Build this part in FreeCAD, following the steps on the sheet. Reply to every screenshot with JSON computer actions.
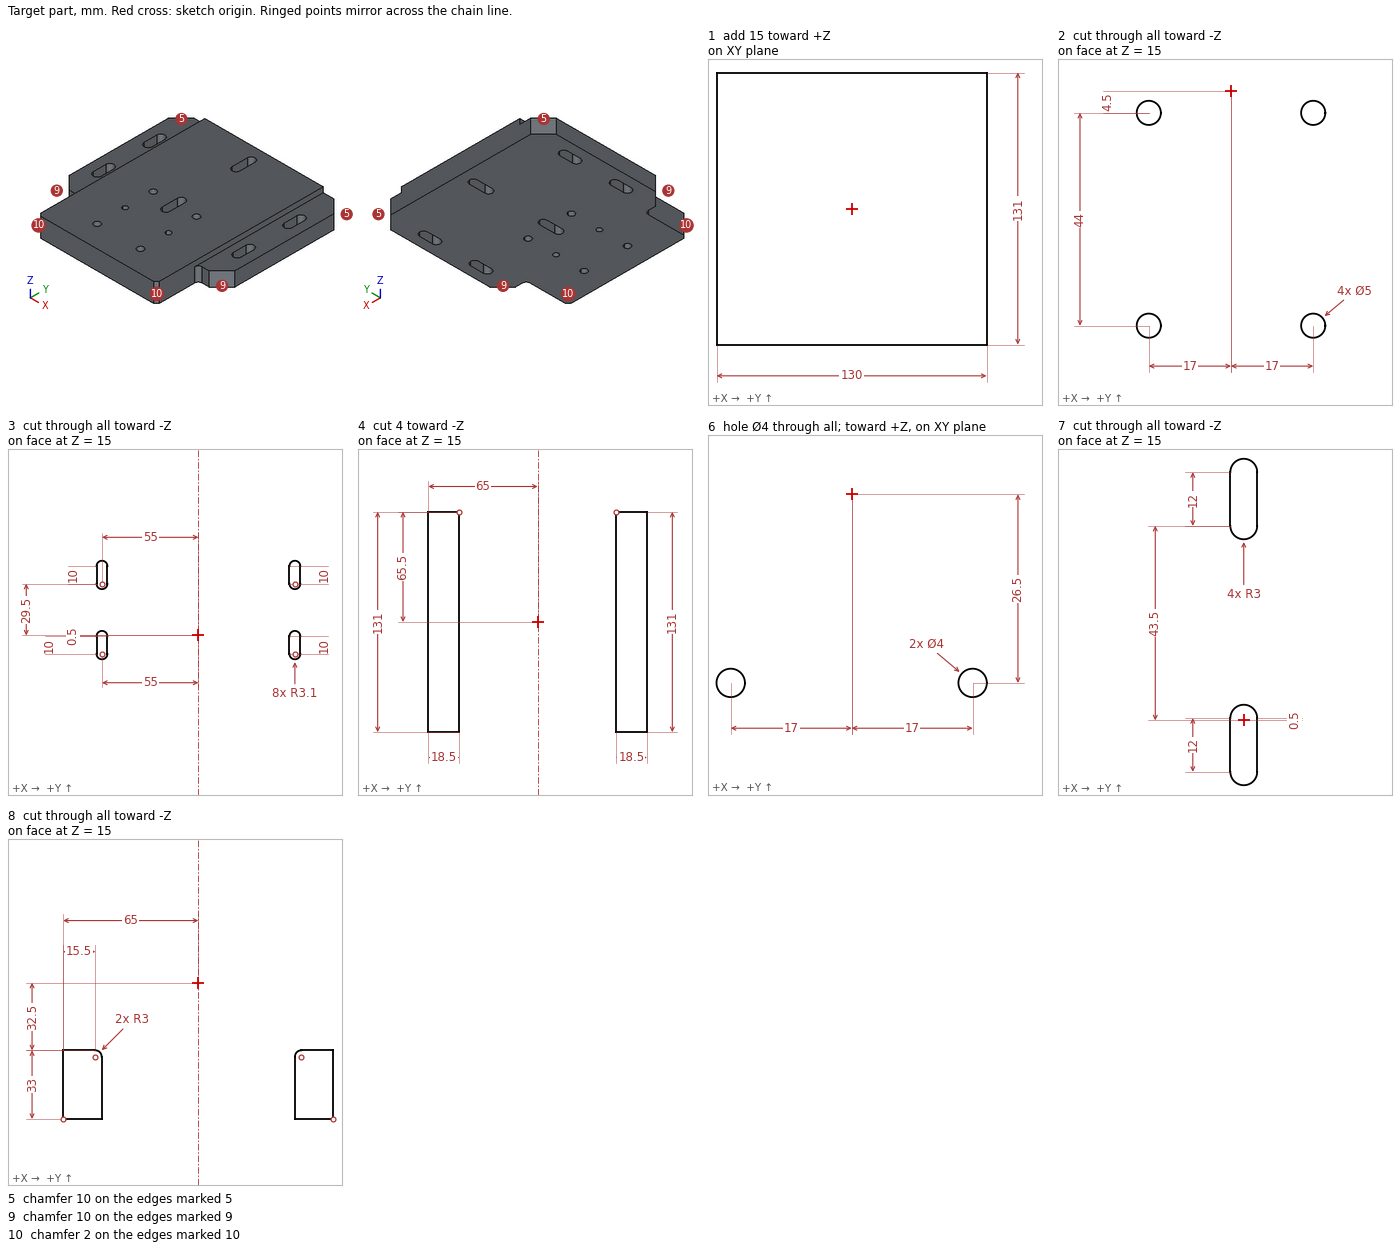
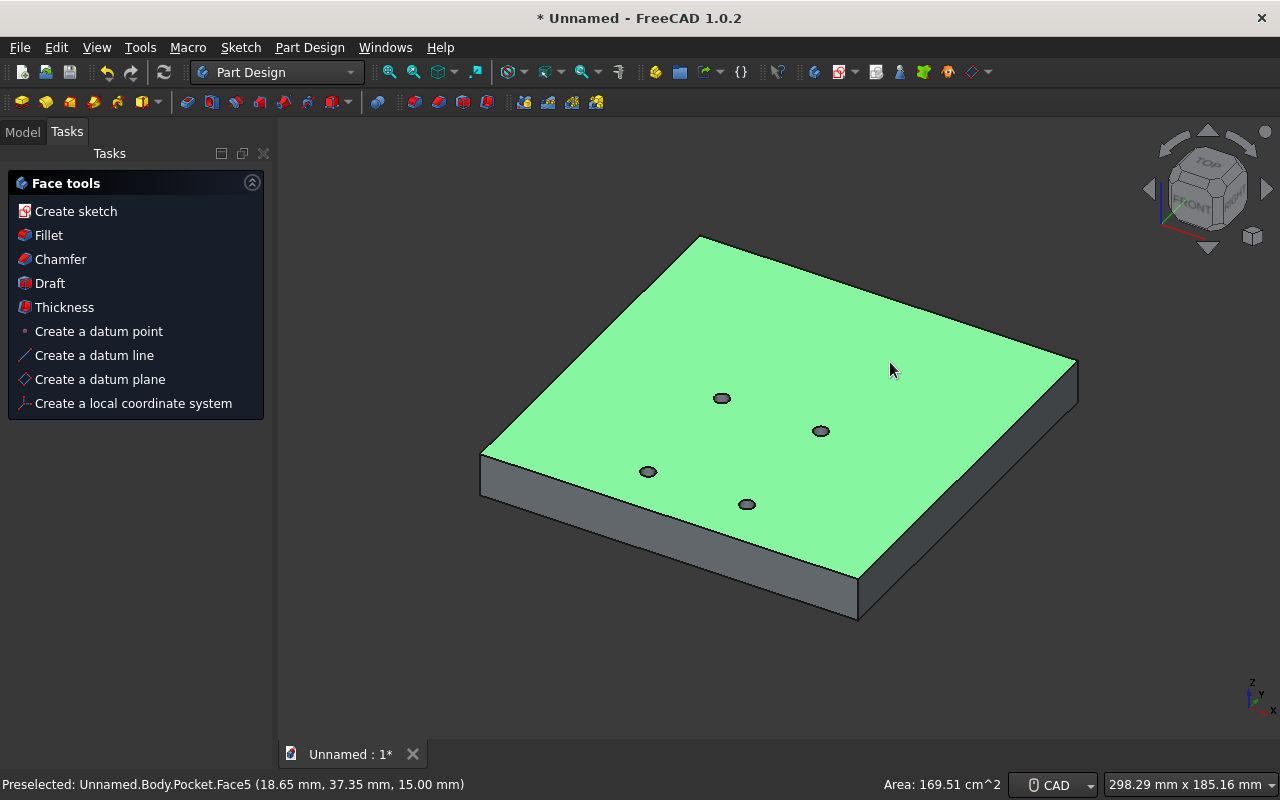
{"action": "left_click", "coordinate": [840, 72]}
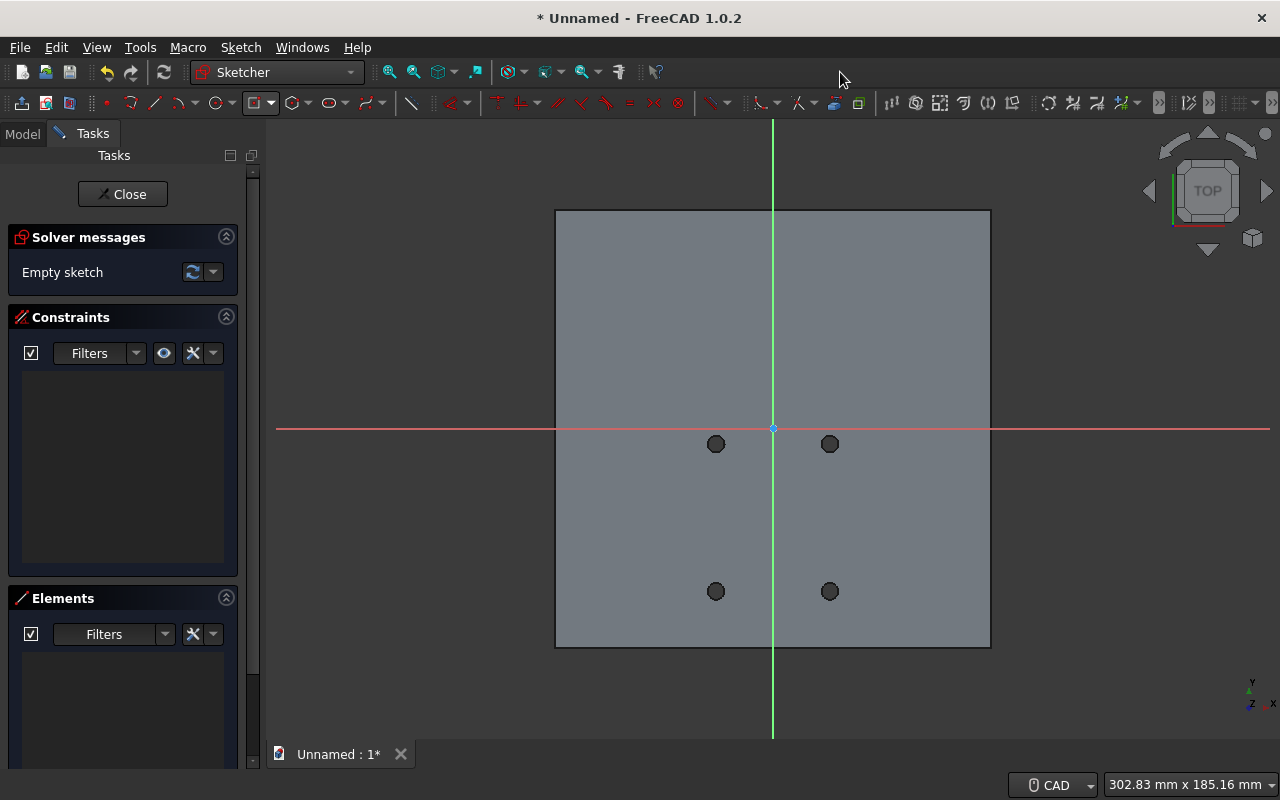
{"action": "scroll", "coordinate": [912, 282], "scroll_direction": "up", "scroll_amount": 2}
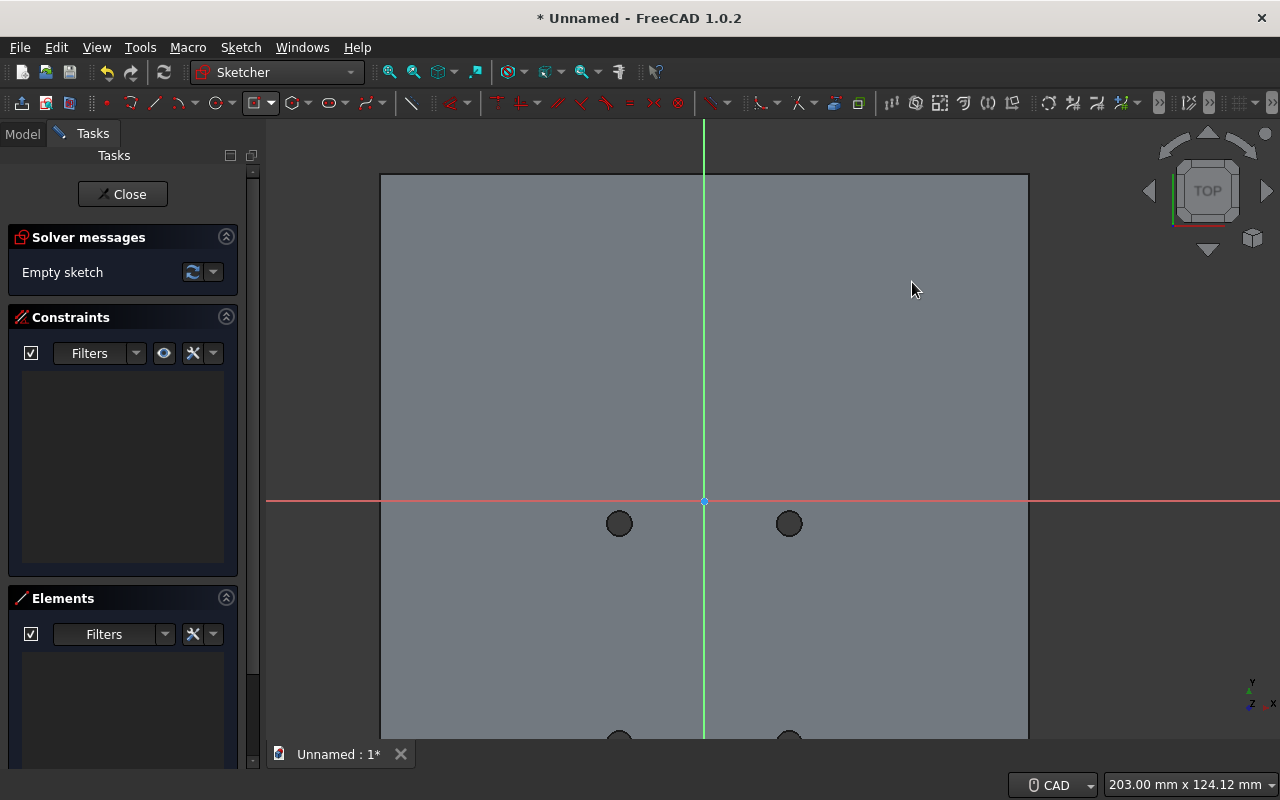
{"action": "left_click", "coordinate": [330, 104]}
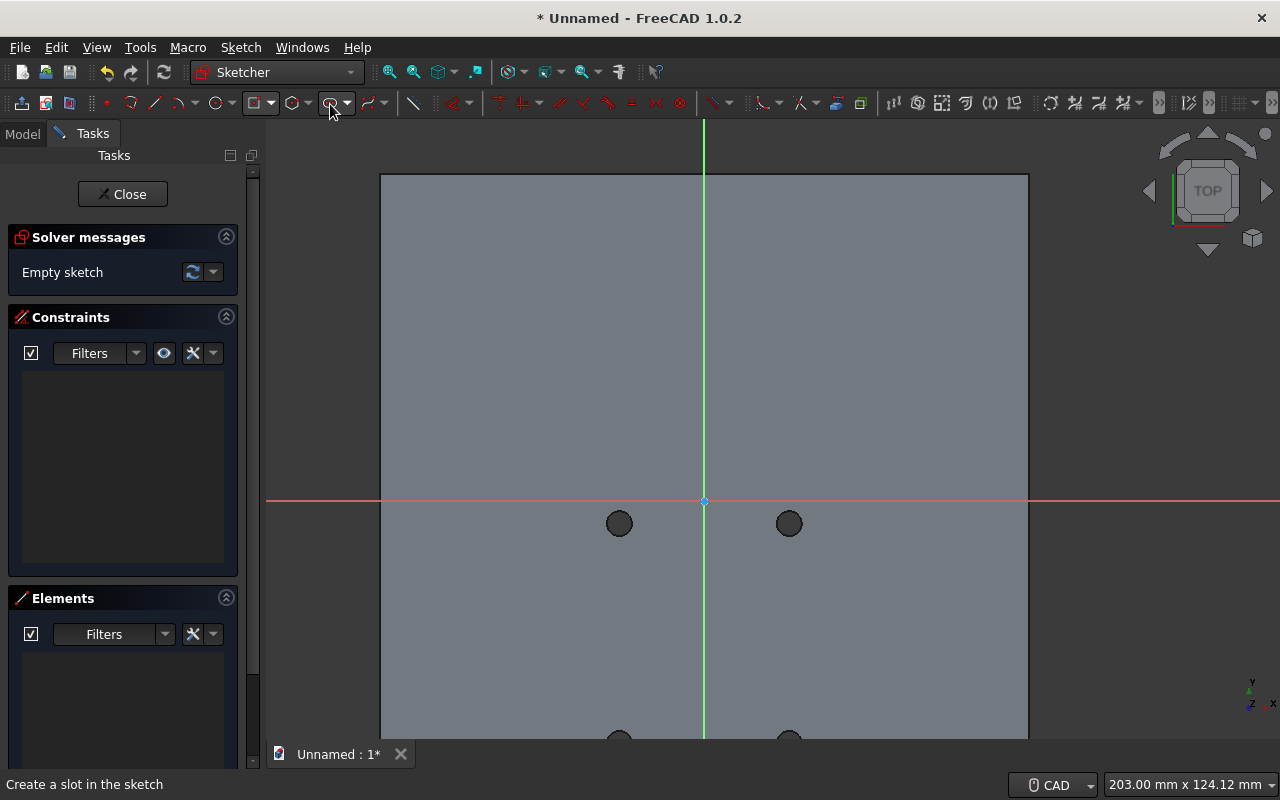
{"action": "scroll", "coordinate": [430, 554], "scroll_direction": "up", "scroll_amount": 2}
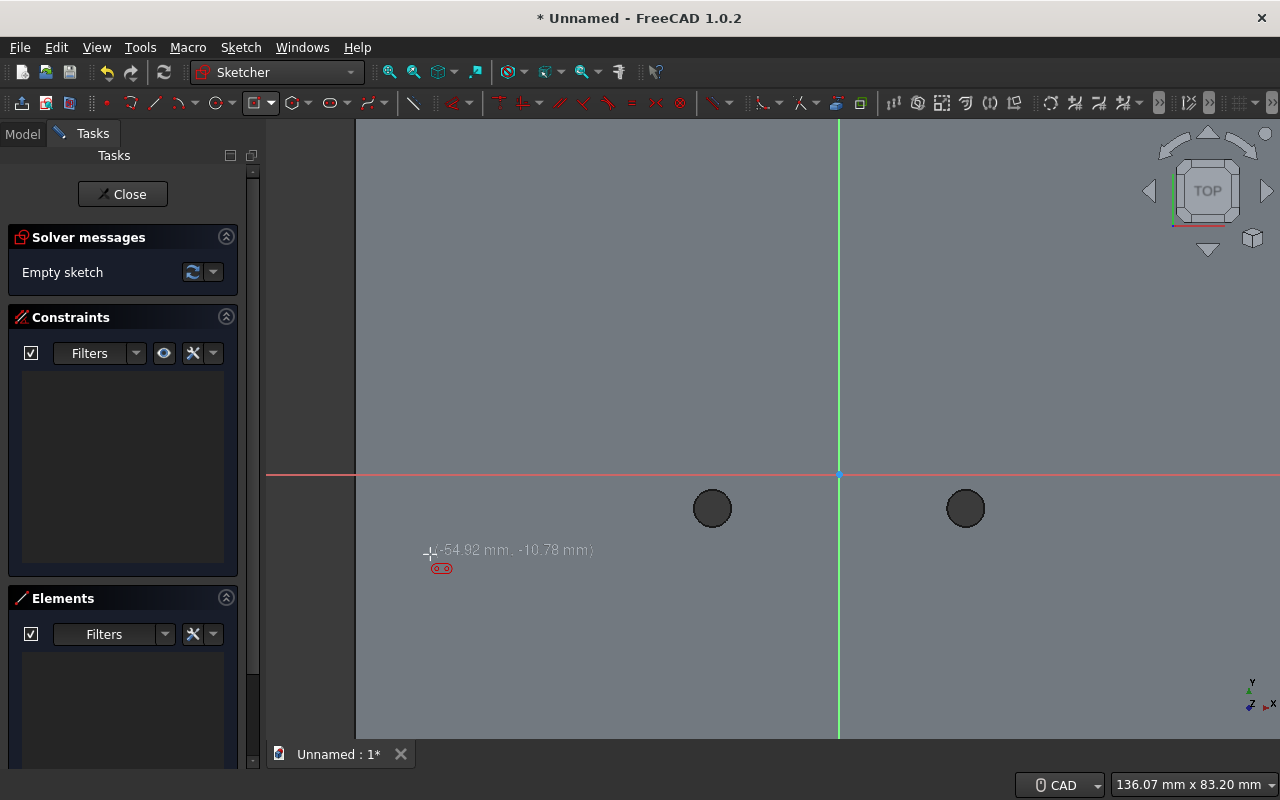
{"action": "left_click", "coordinate": [429, 553]}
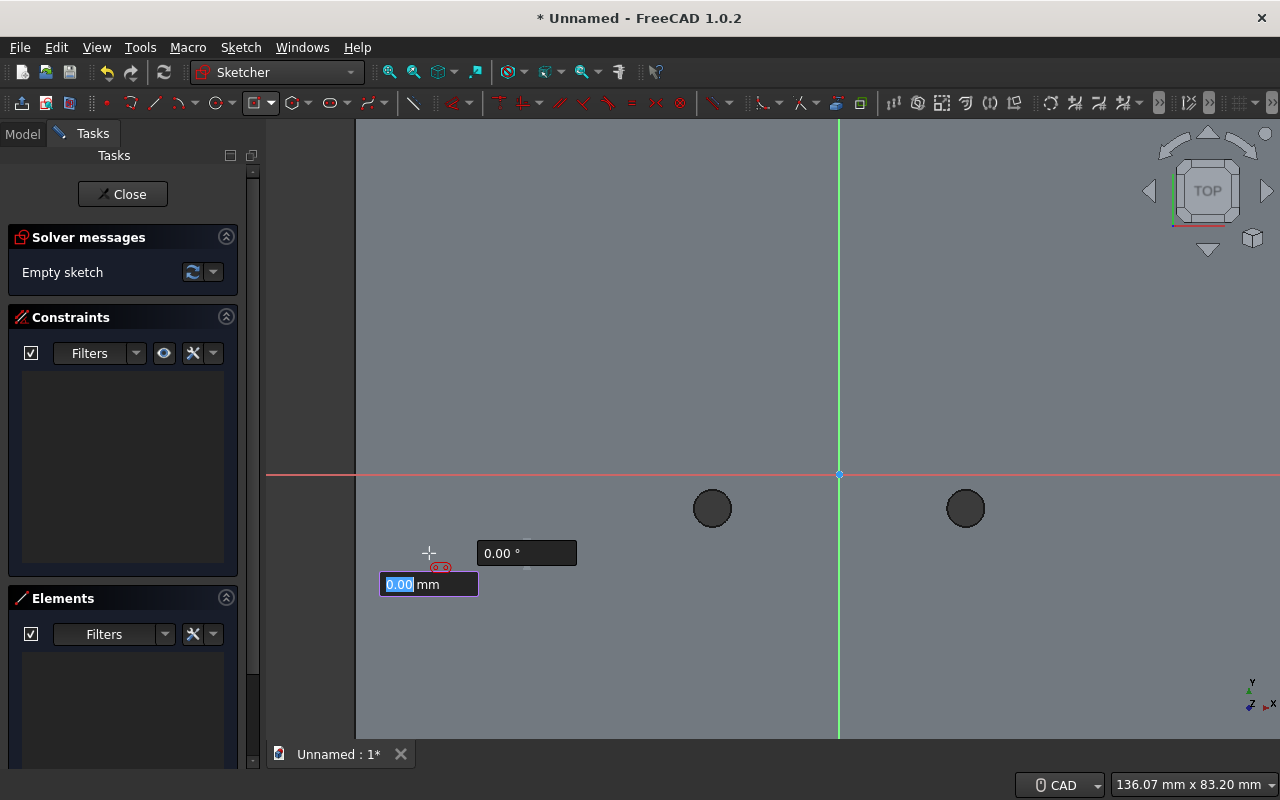
{"action": "scroll", "coordinate": [429, 479], "scroll_direction": "up", "scroll_amount": 8}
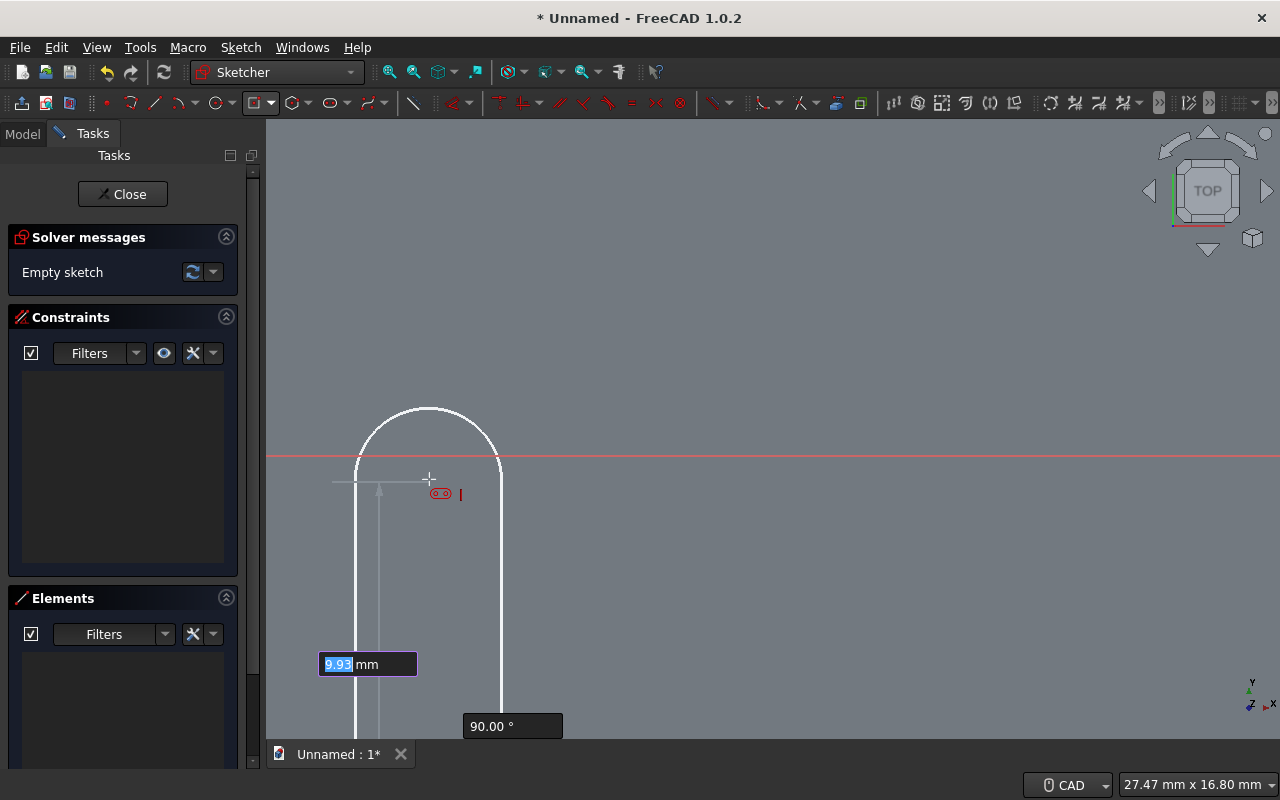
{"action": "left_click", "coordinate": [428, 475]}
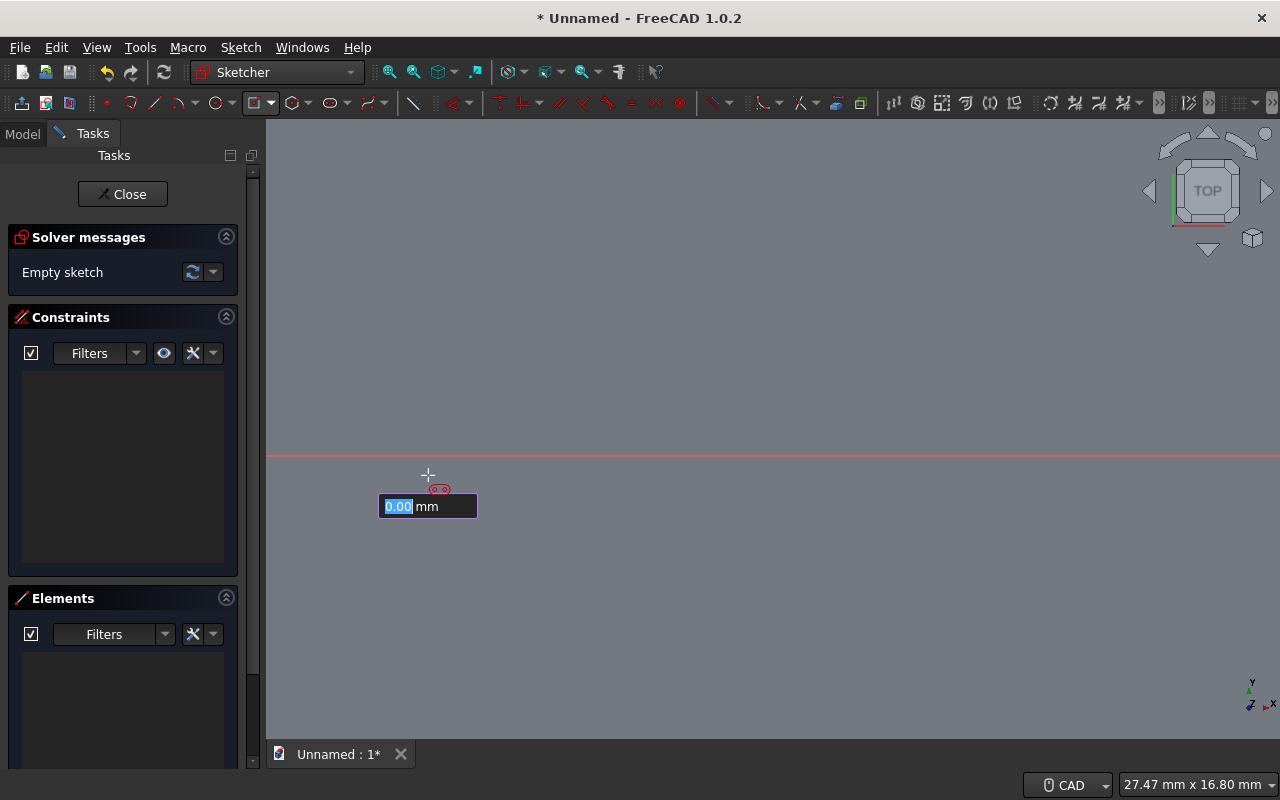
{"action": "scroll", "coordinate": [430, 509], "scroll_direction": "down", "scroll_amount": 10}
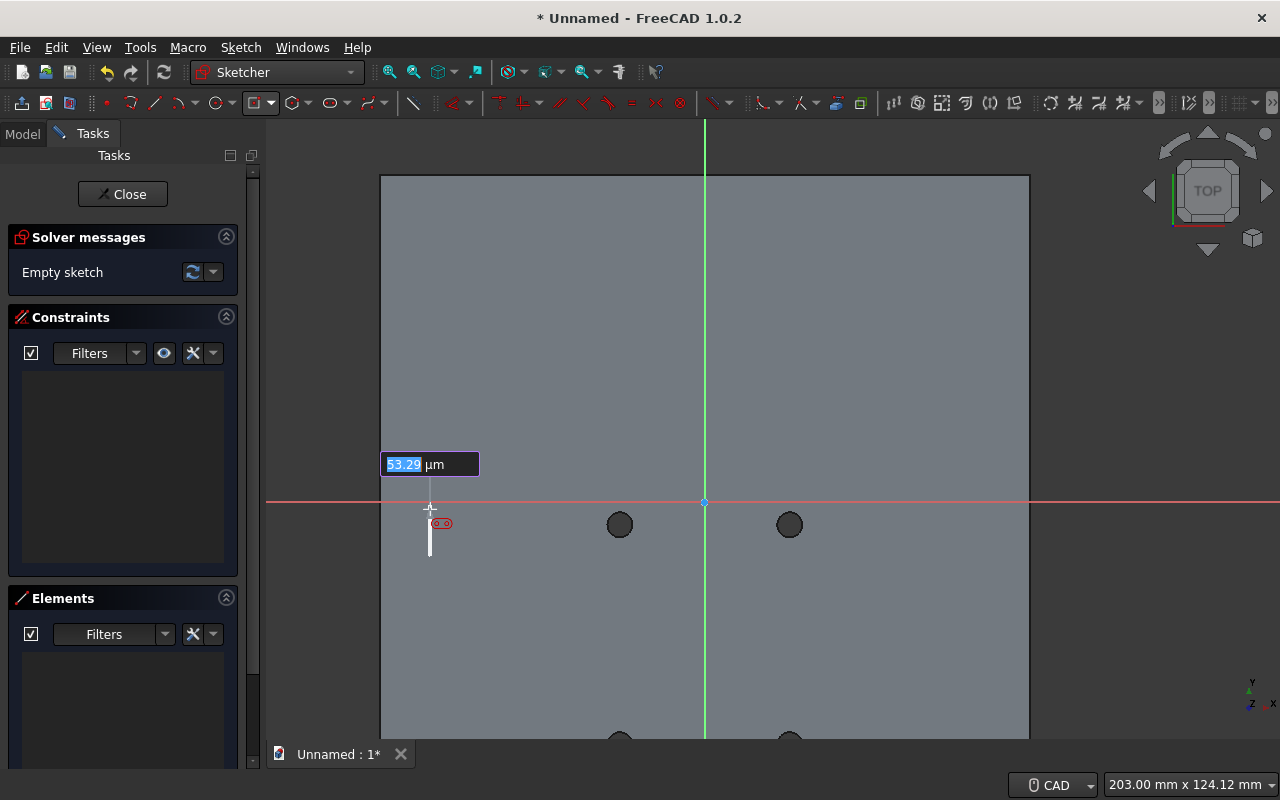
{"action": "left_click", "coordinate": [415, 530]}